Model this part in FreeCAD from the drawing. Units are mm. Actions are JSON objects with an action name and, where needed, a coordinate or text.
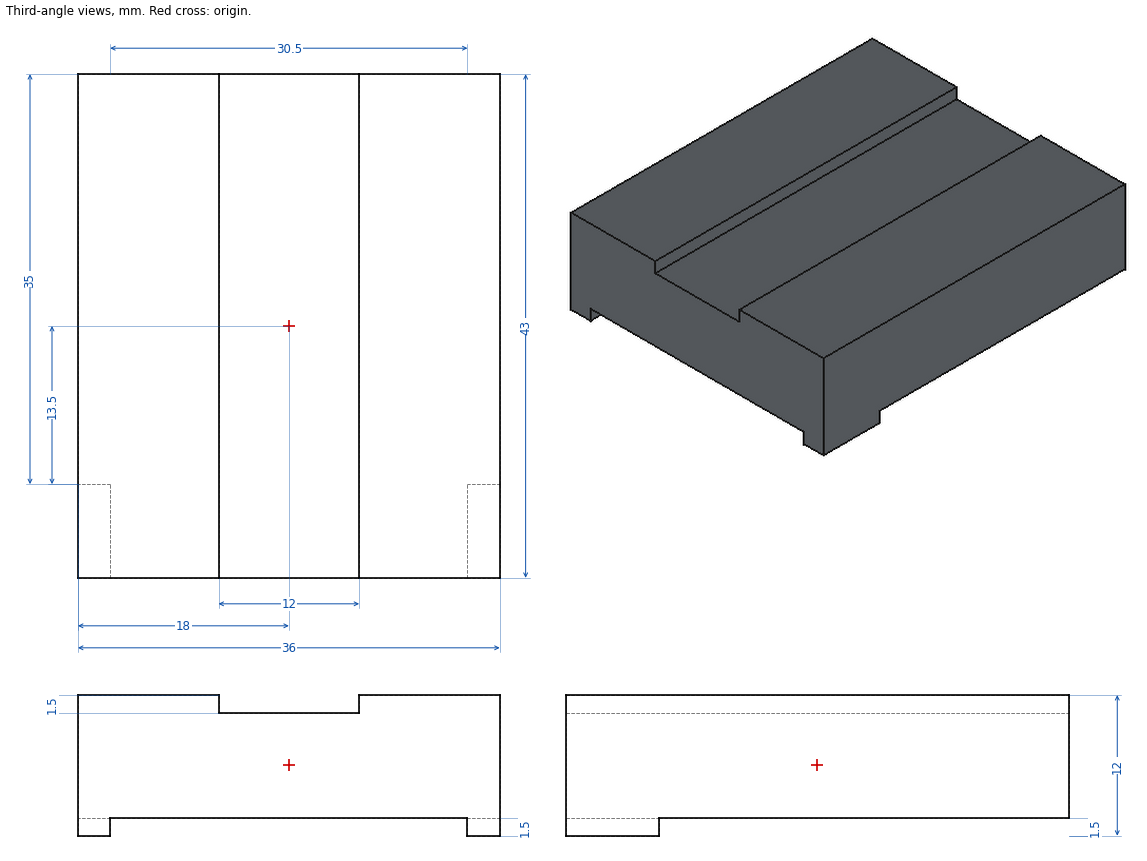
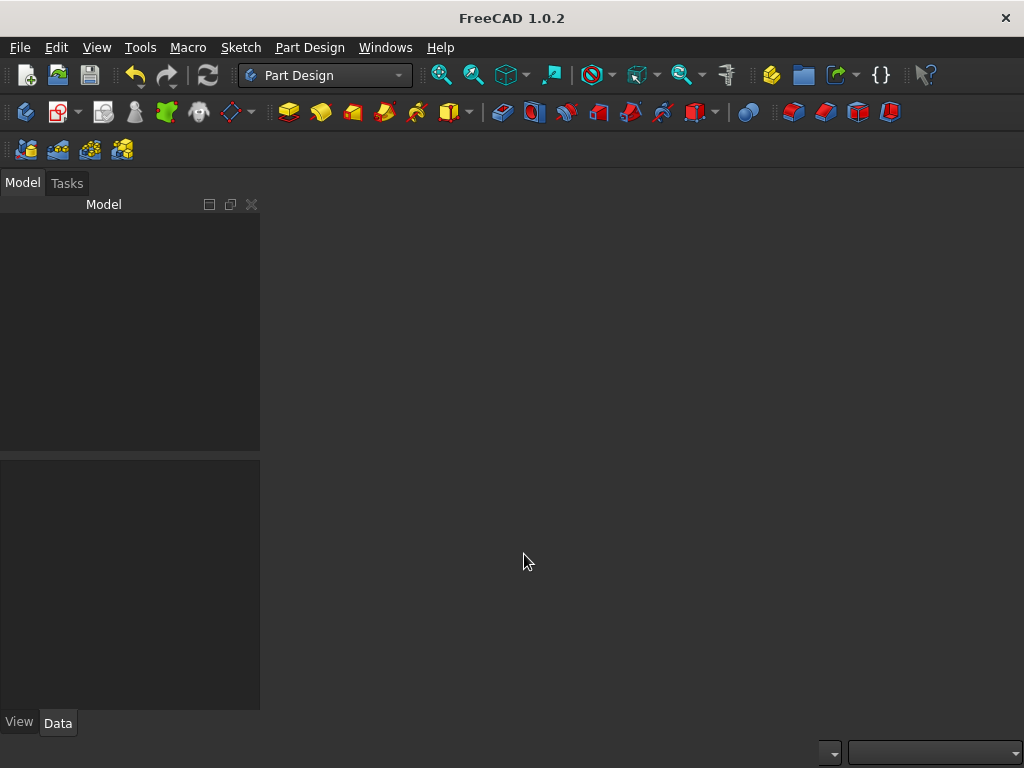
{"action": "key", "text": "ctrl+n"}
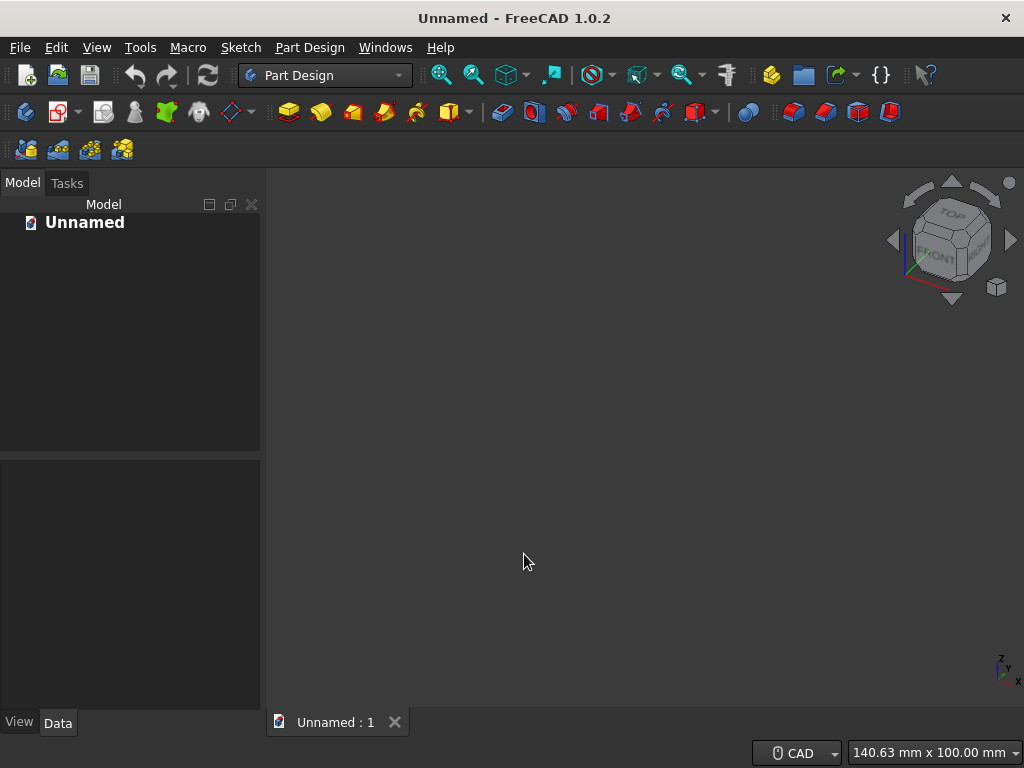
{"action": "left_click", "coordinate": [58, 112]}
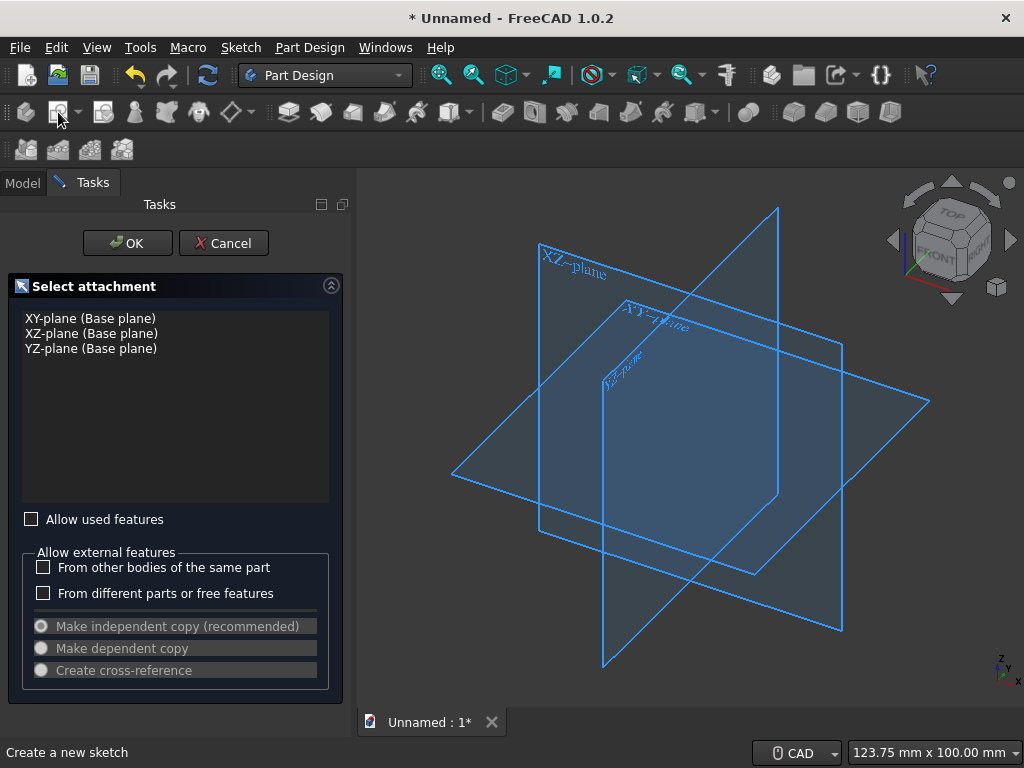
{"action": "left_click", "coordinate": [82, 318]}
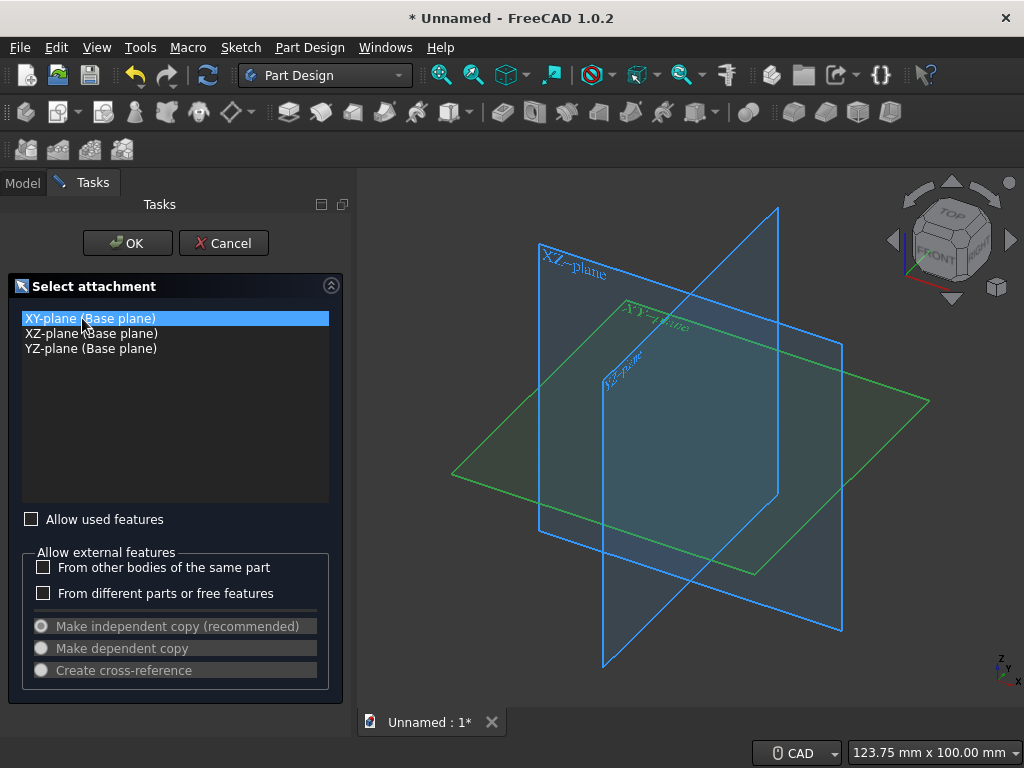
{"action": "left_click", "coordinate": [128, 243]}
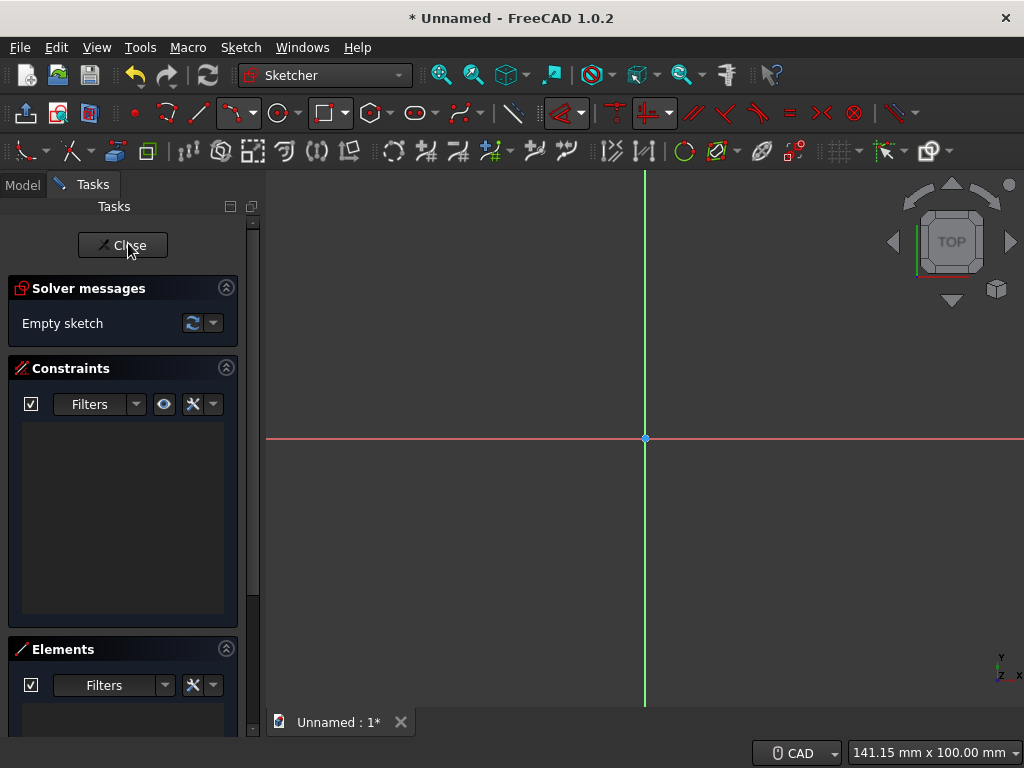
{"action": "scroll", "coordinate": [784, 439], "scroll_direction": "up", "scroll_amount": 2}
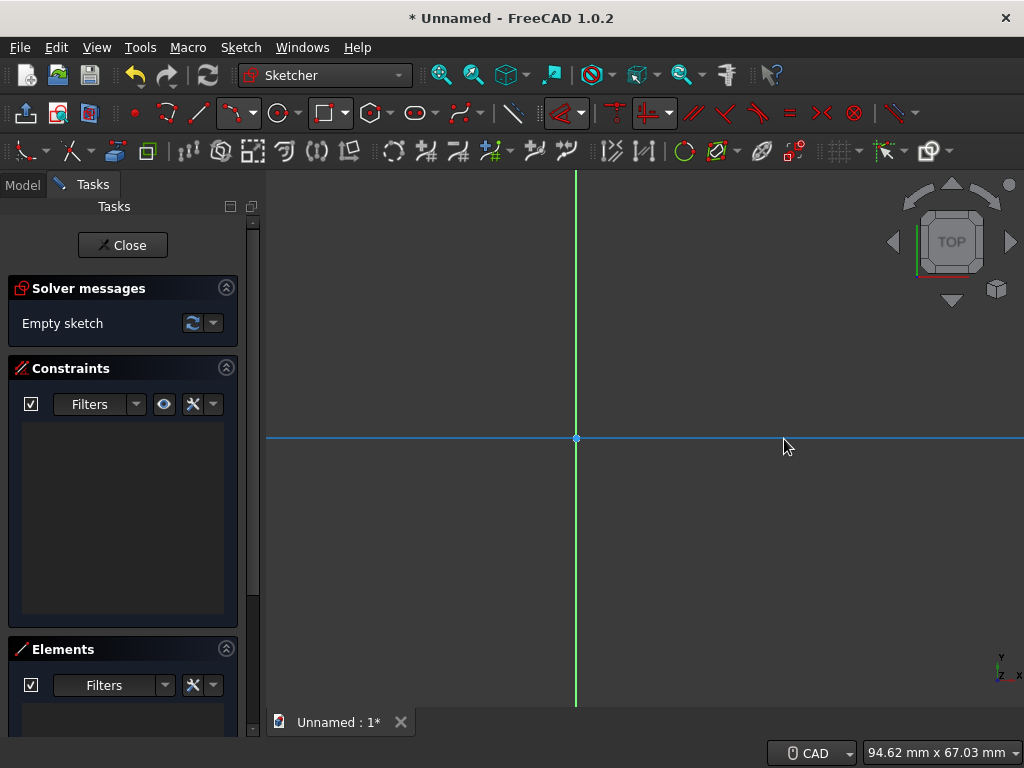
{"action": "key", "text": "g v"}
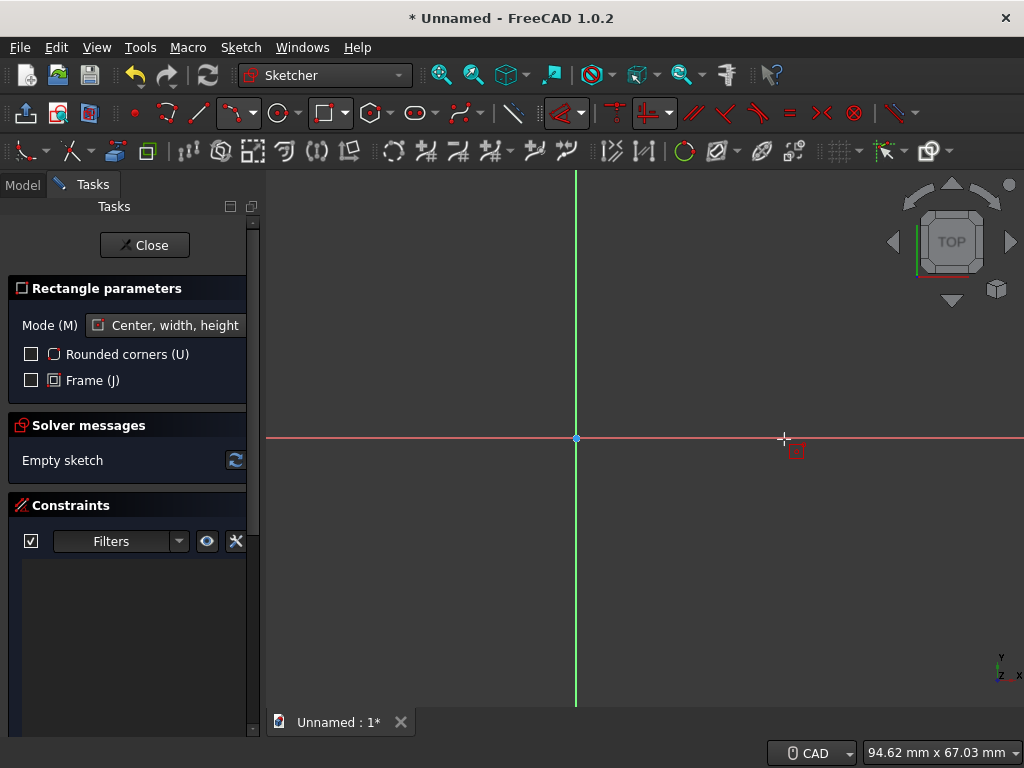
{"action": "left_click", "coordinate": [576, 438]}
{"action": "left_click", "coordinate": [720, 266]}
{"action": "key", "text": "Escape"}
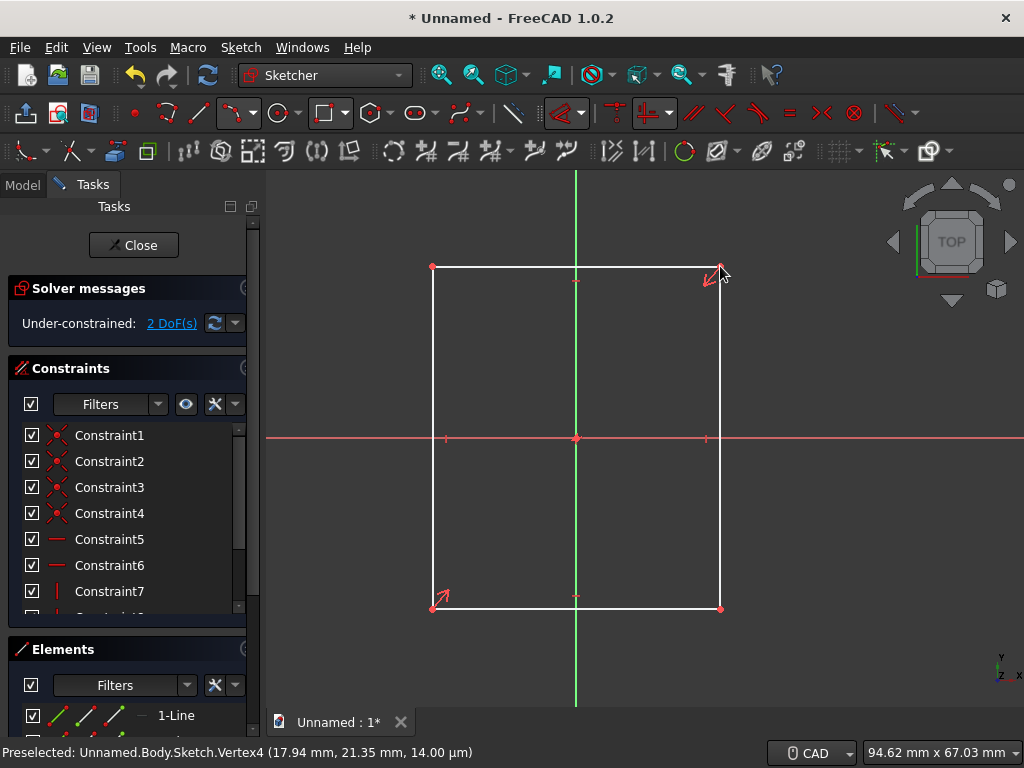
{"action": "key", "text": "d"}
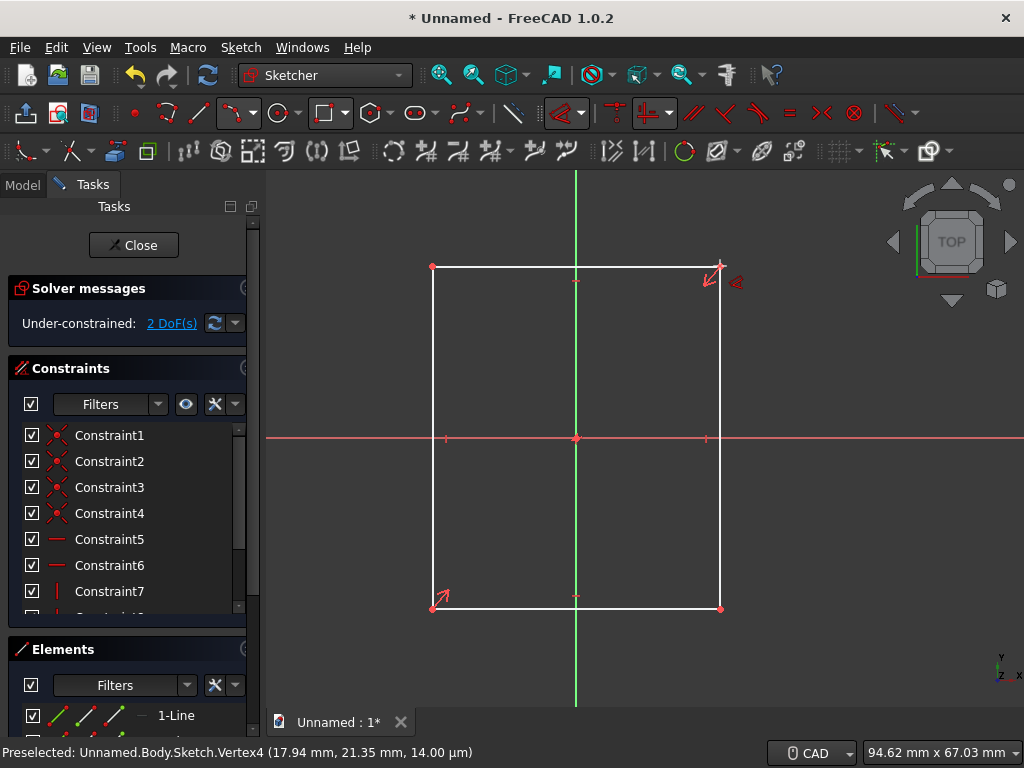
{"action": "left_click", "coordinate": [519, 609]}
{"action": "left_click", "coordinate": [510, 643]}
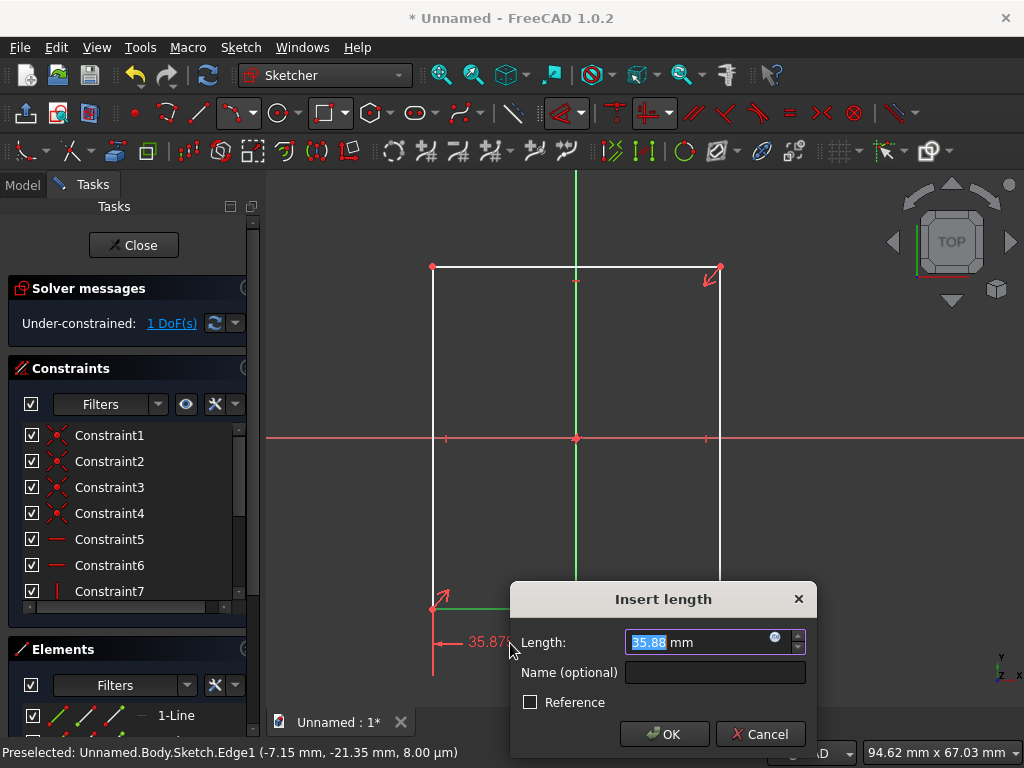
{"action": "type", "text": "36"}
{"action": "key", "text": "Return"}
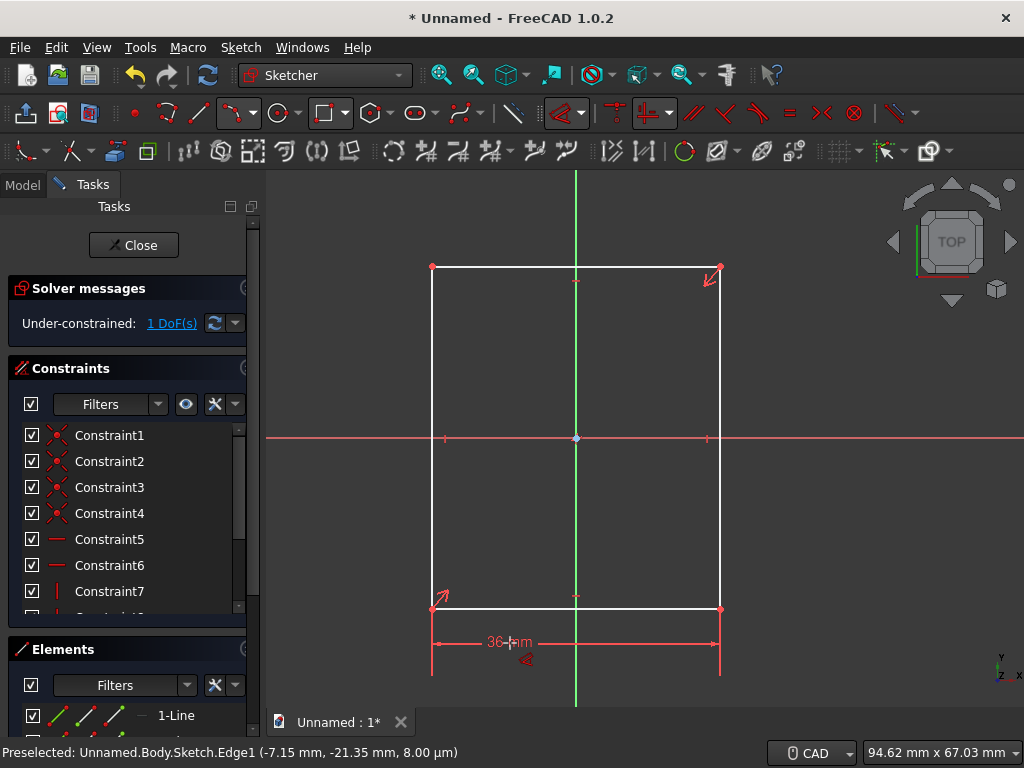
{"action": "left_click", "coordinate": [720, 506]}
{"action": "left_click", "coordinate": [754, 359]}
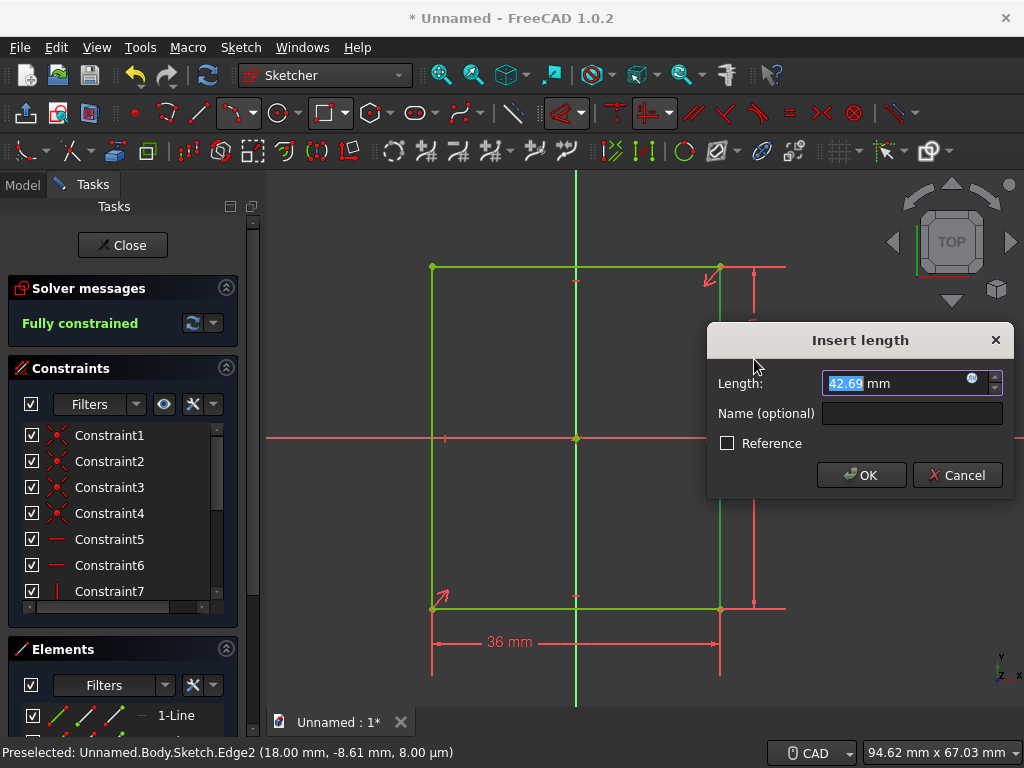
{"action": "type", "text": "43"}
{"action": "key", "text": "Return"}
{"action": "key", "text": "Escape"}